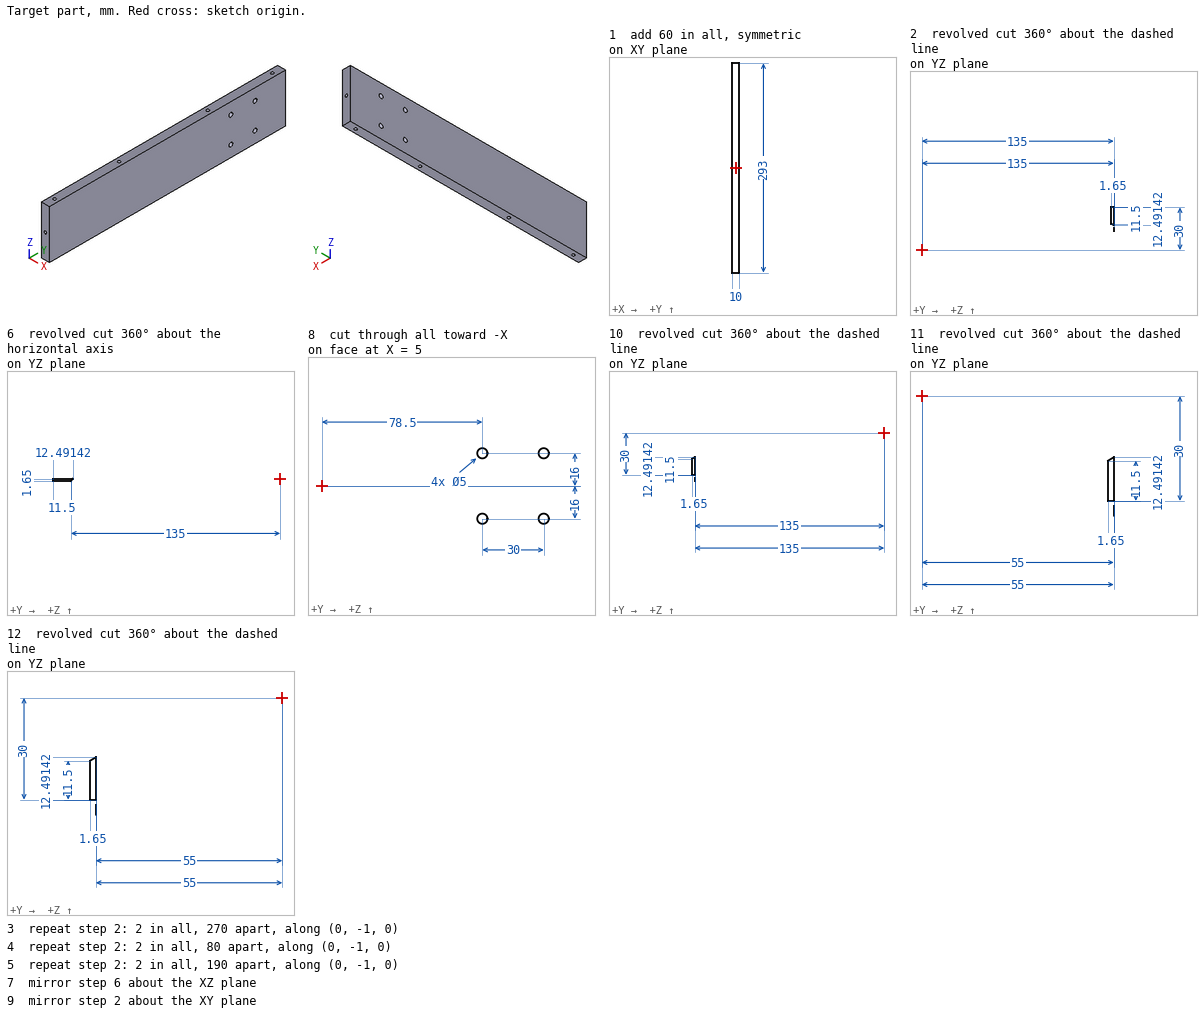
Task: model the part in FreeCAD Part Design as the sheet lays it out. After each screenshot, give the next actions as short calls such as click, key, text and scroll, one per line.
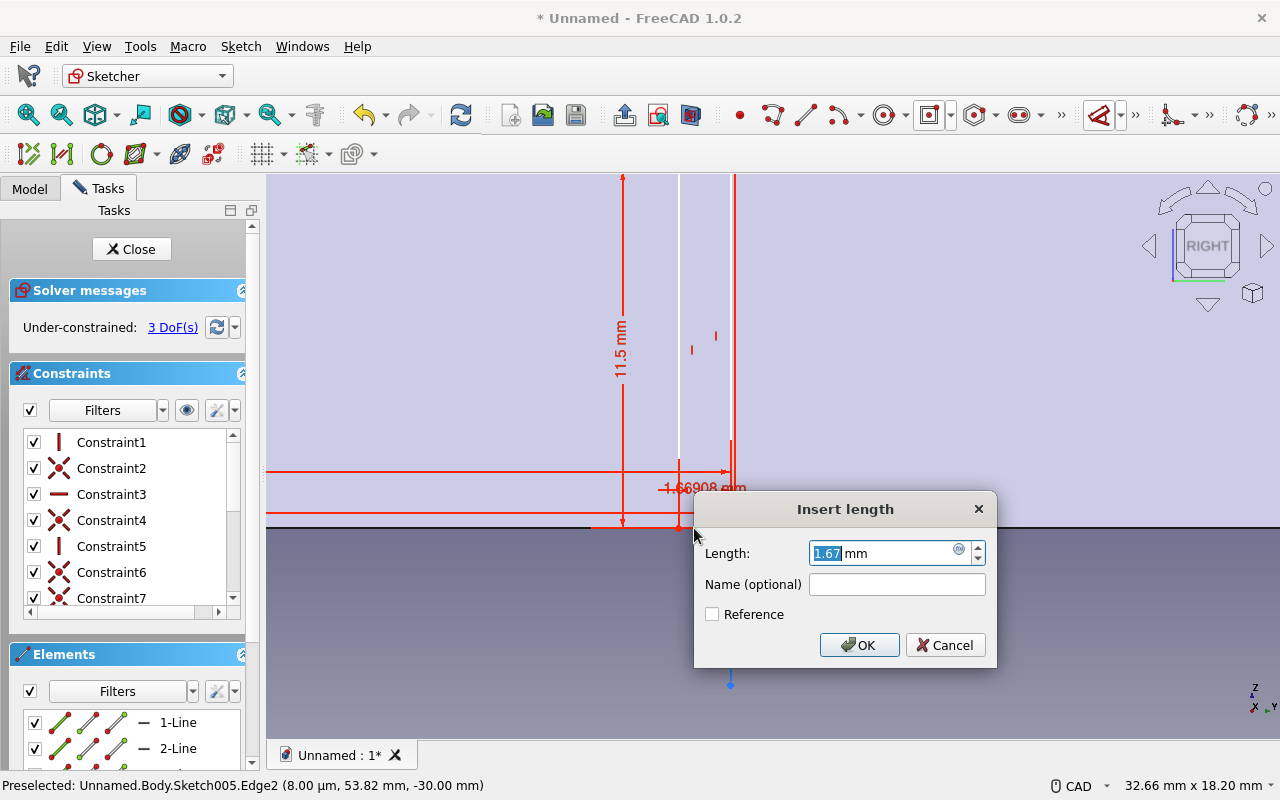
text(1.65)
key(Return)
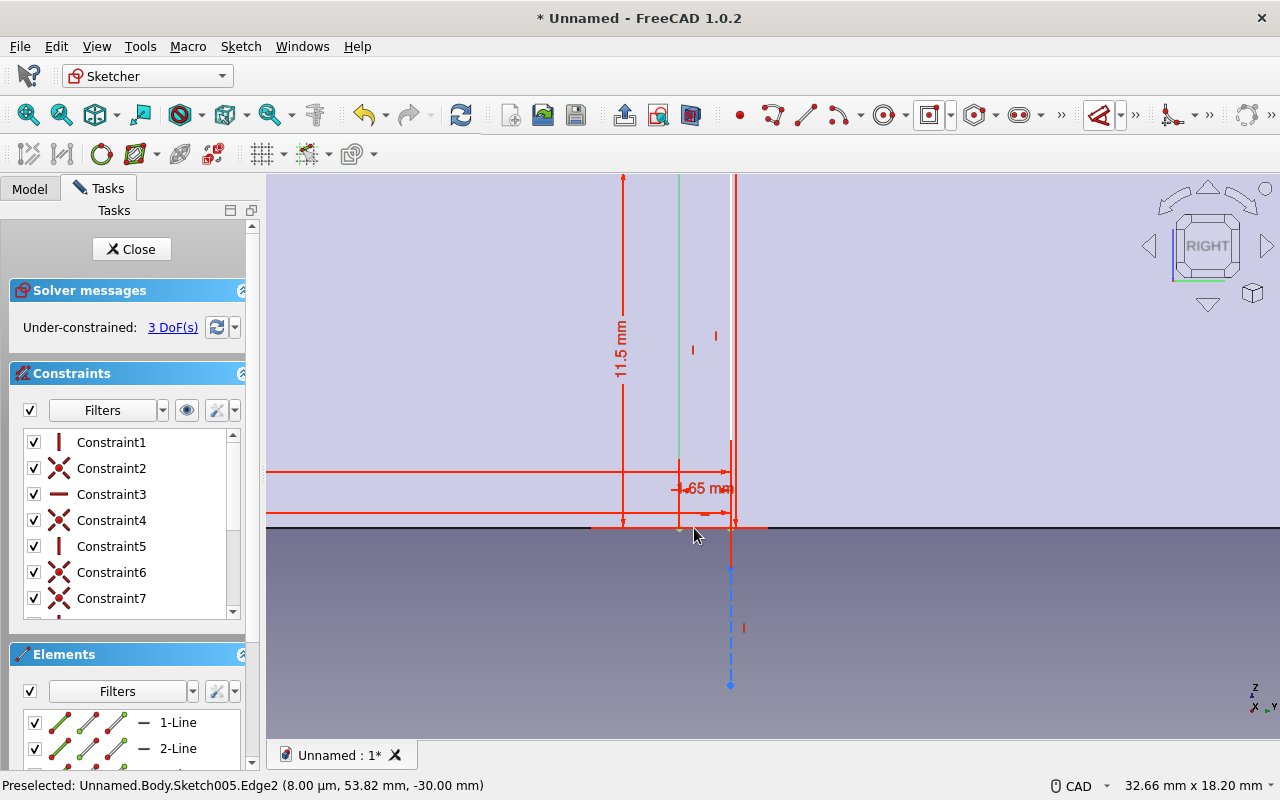
click(731, 412)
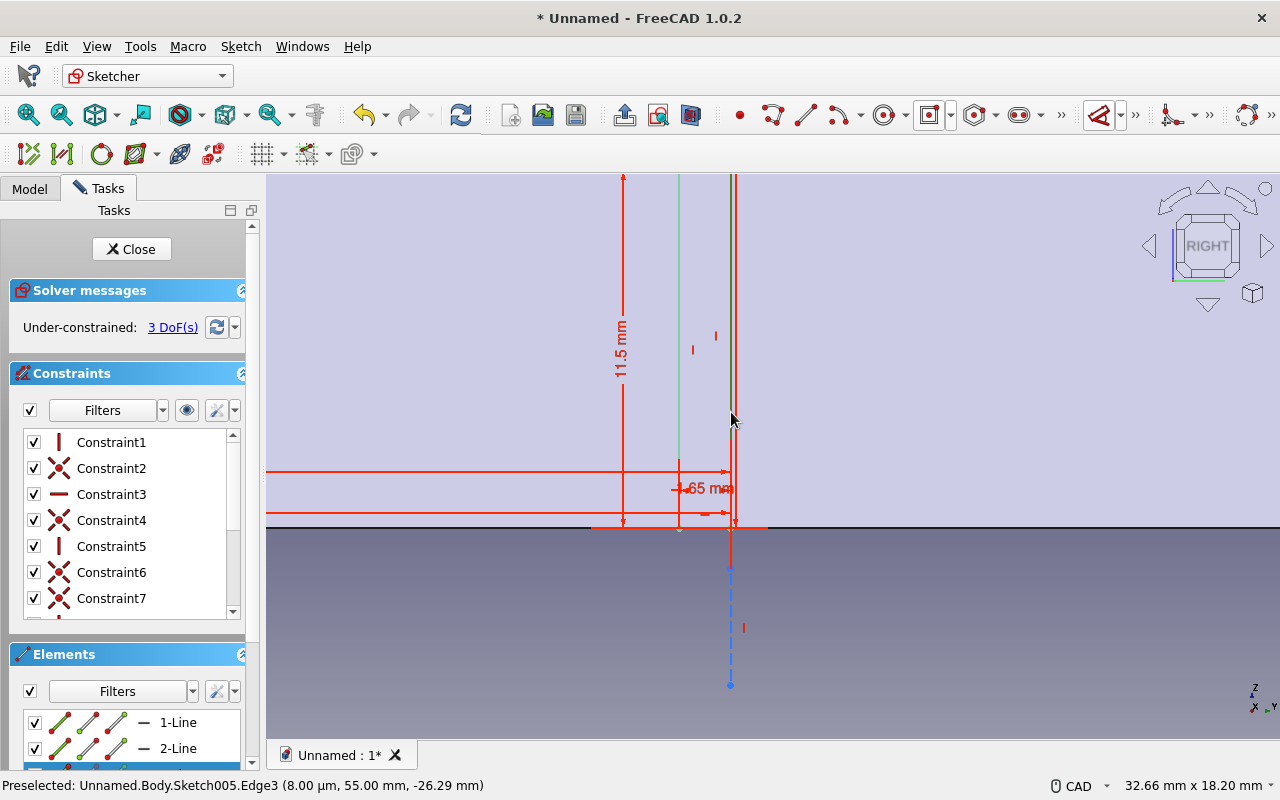
click(1120, 116)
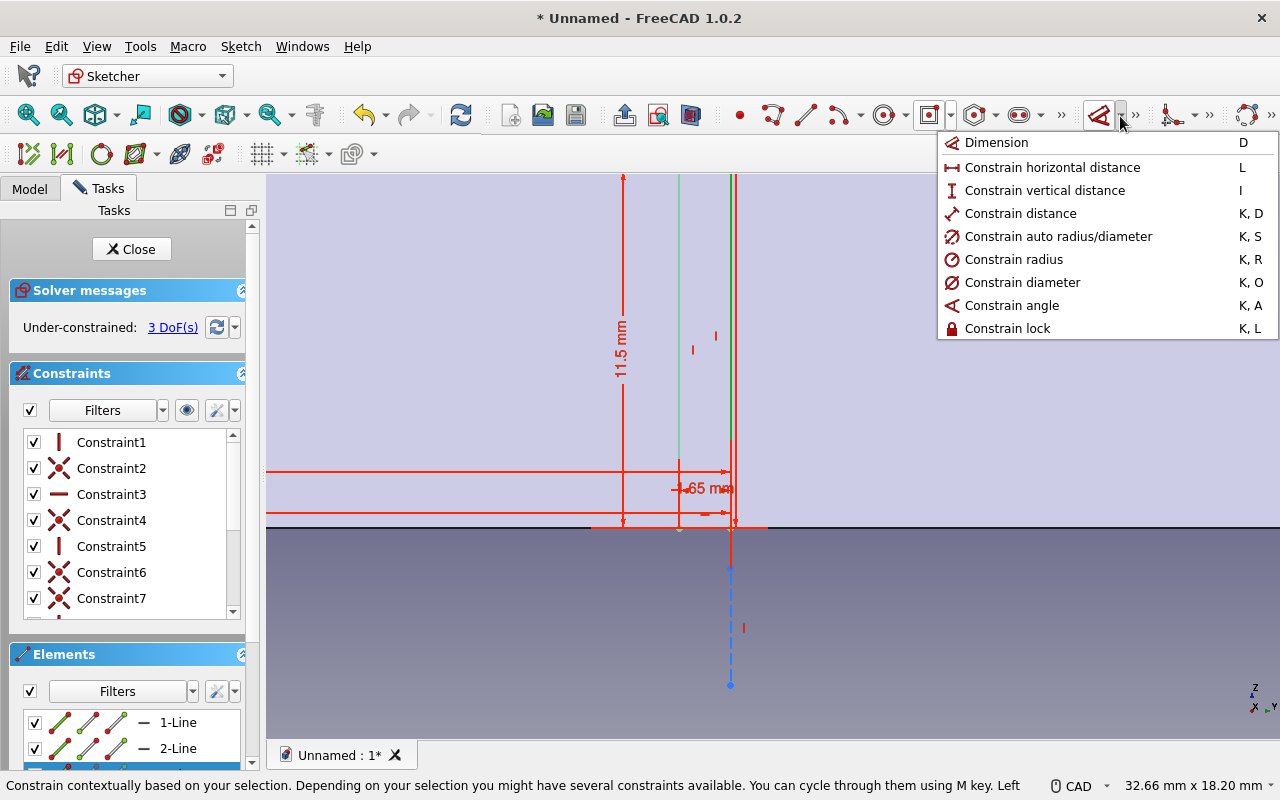
click(1108, 190)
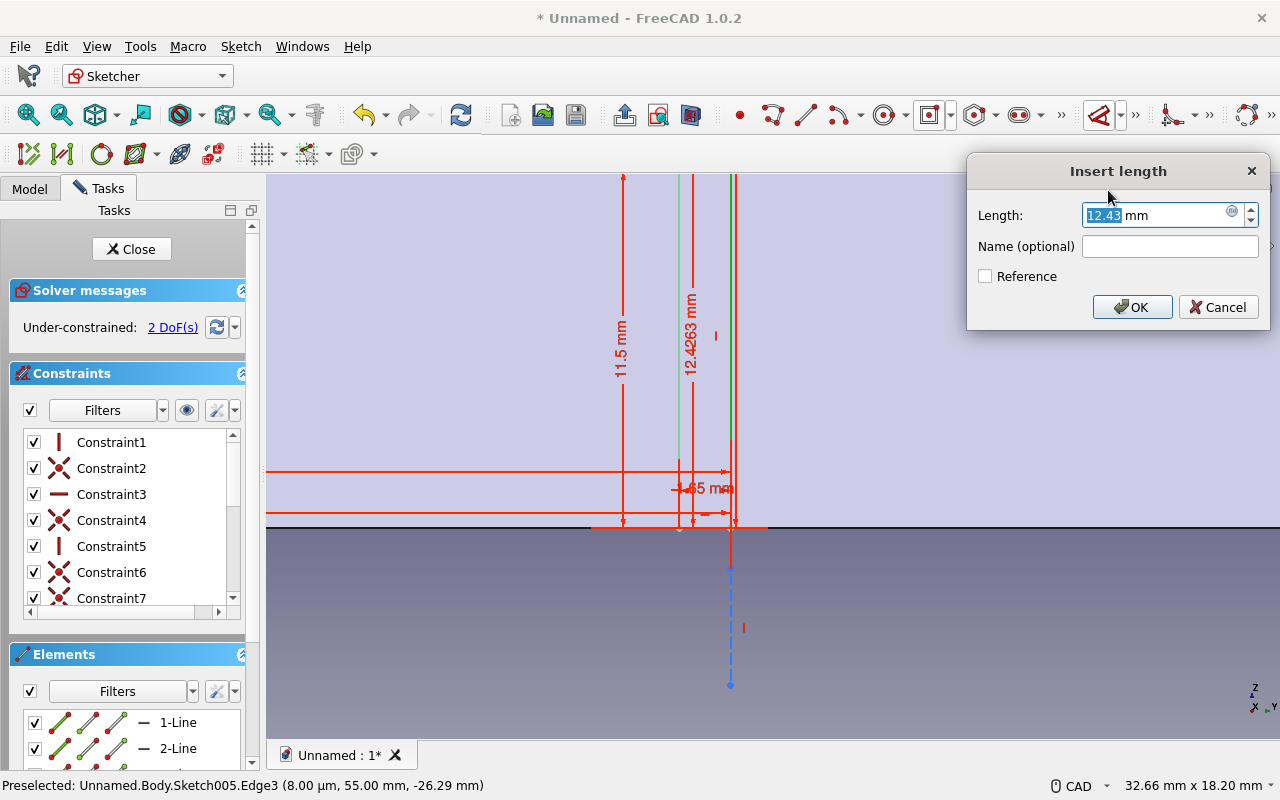
text(12.49142)
key(Return)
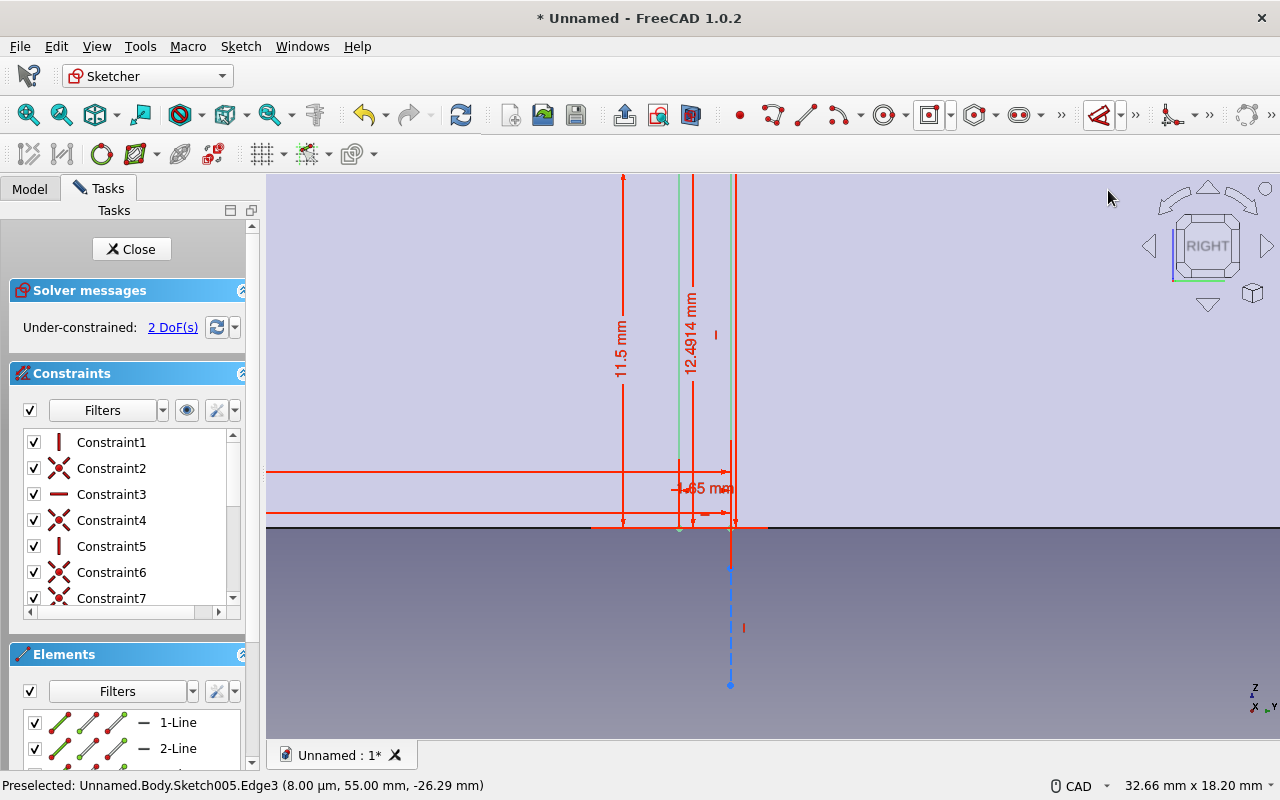
click(132, 249)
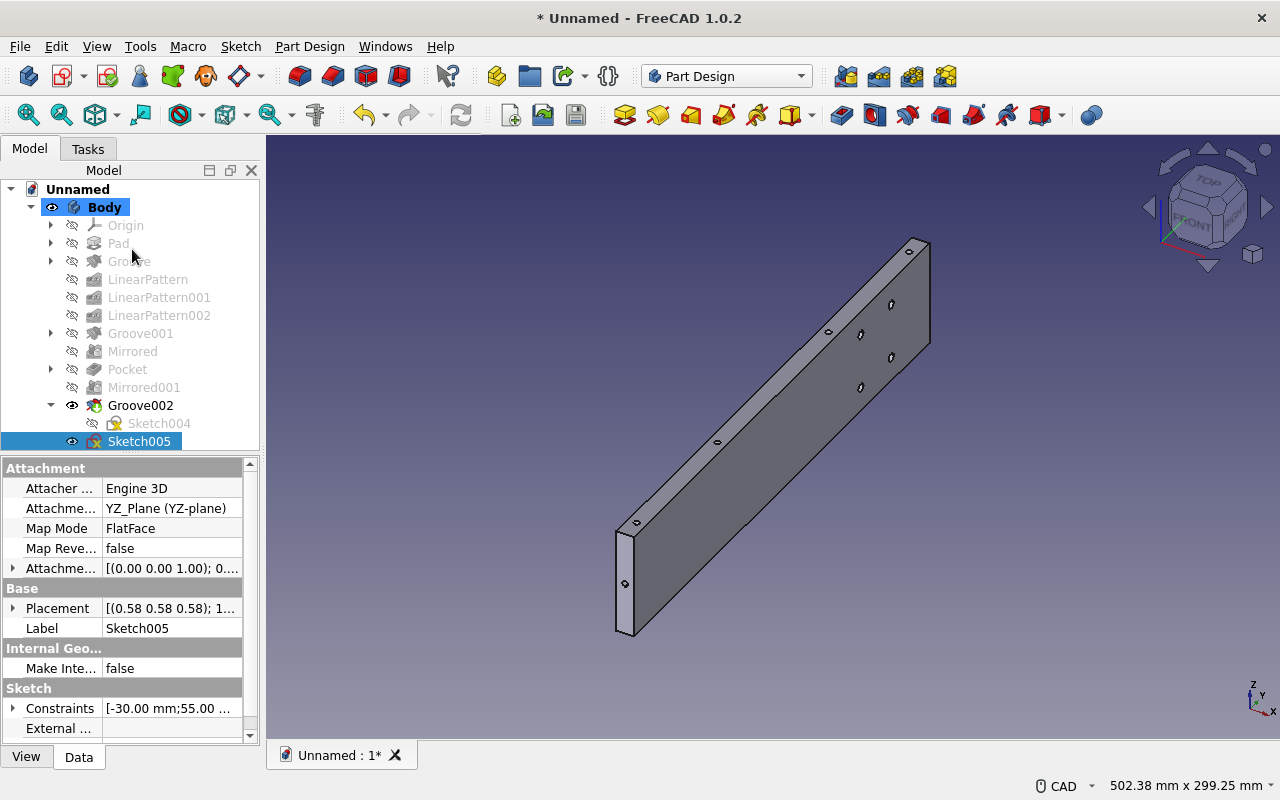
click(908, 116)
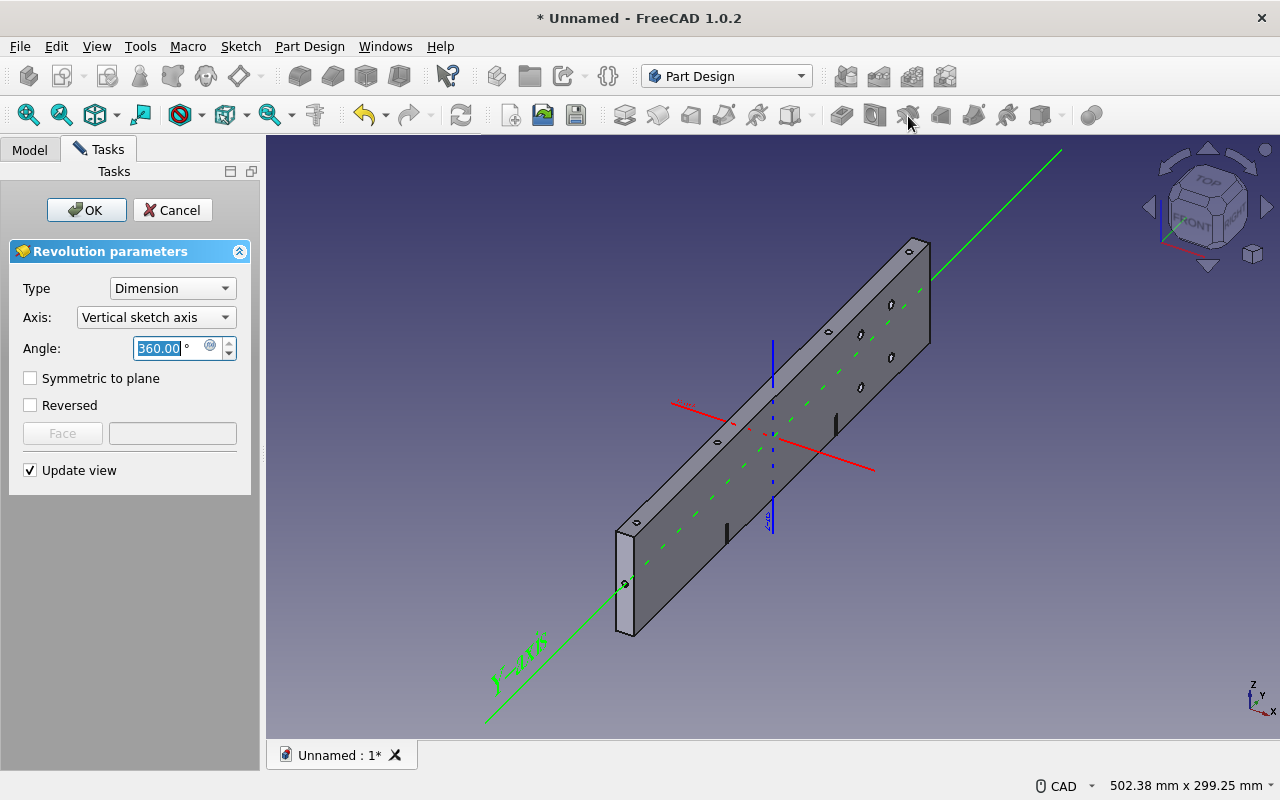
click(157, 318)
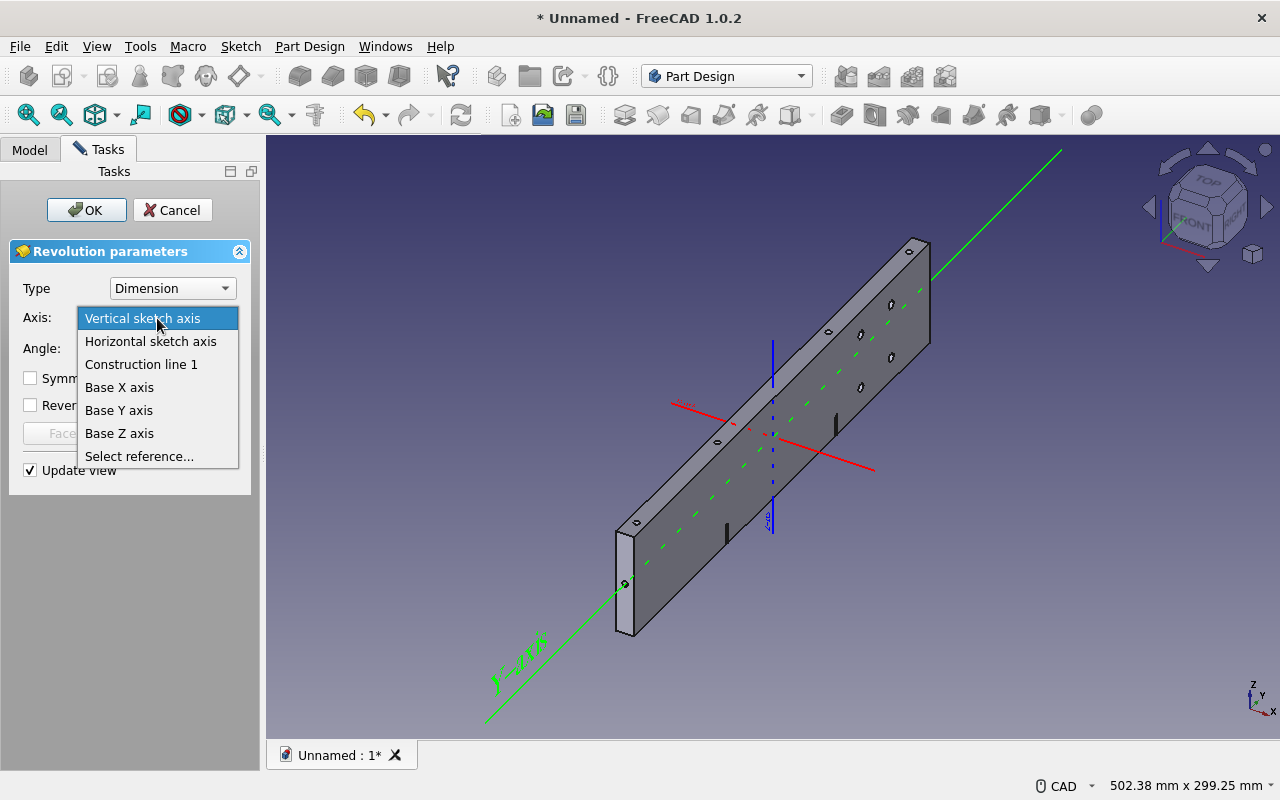
click(156, 364)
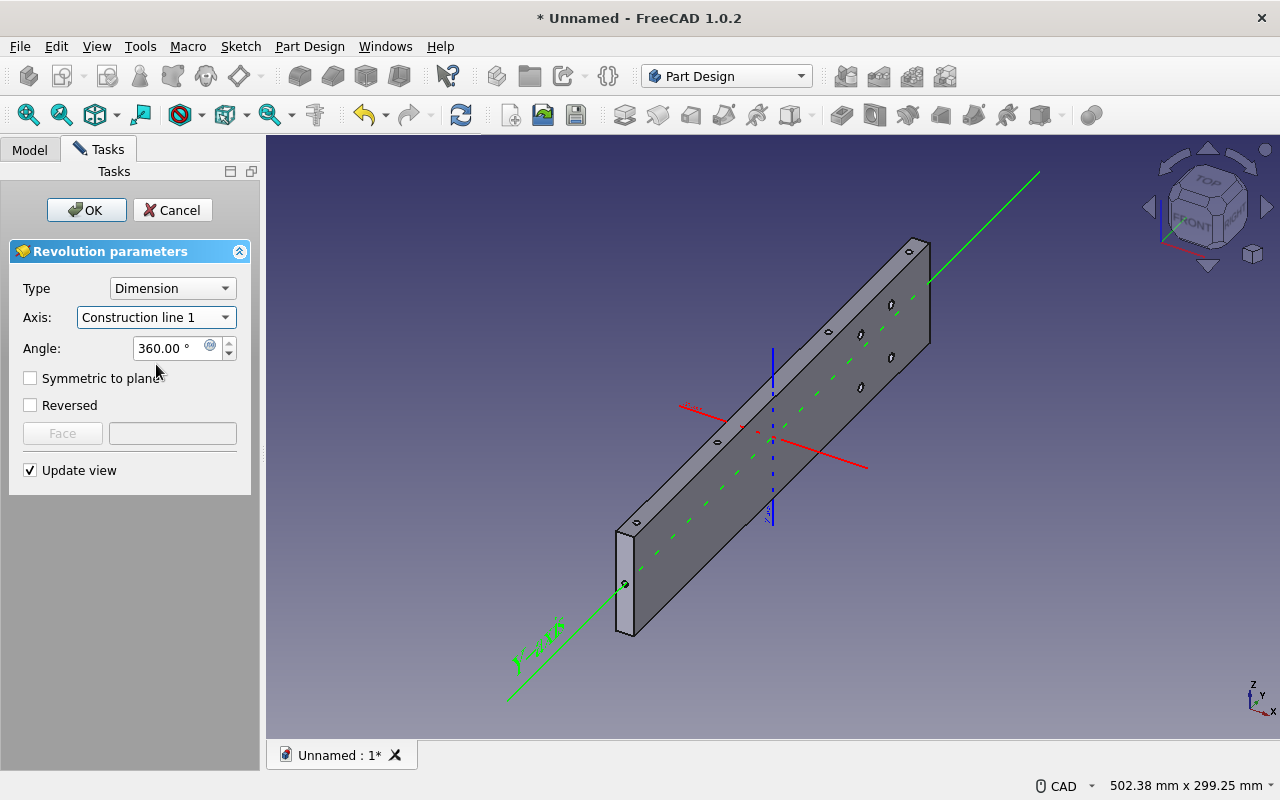
click(87, 210)